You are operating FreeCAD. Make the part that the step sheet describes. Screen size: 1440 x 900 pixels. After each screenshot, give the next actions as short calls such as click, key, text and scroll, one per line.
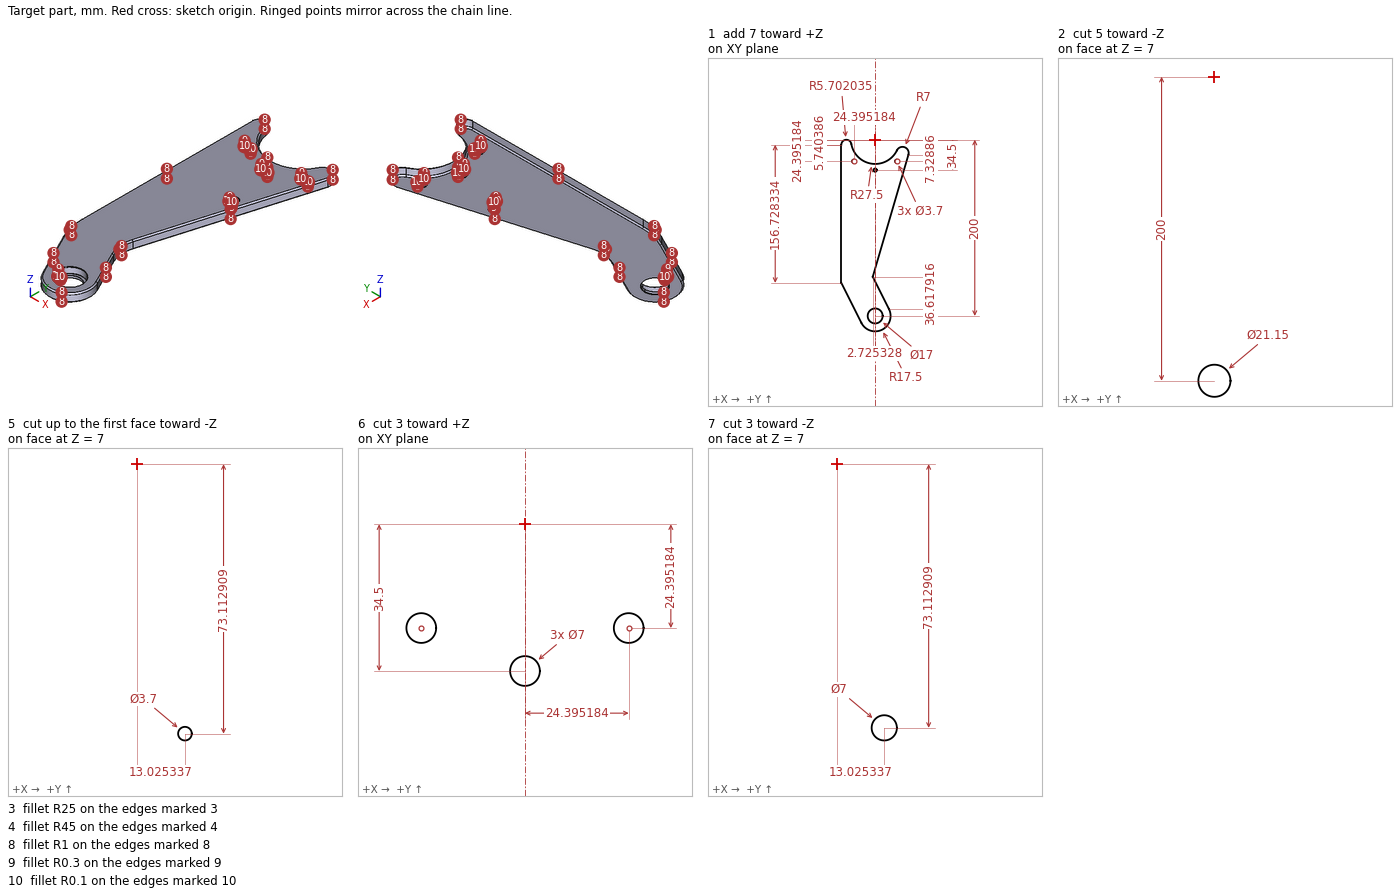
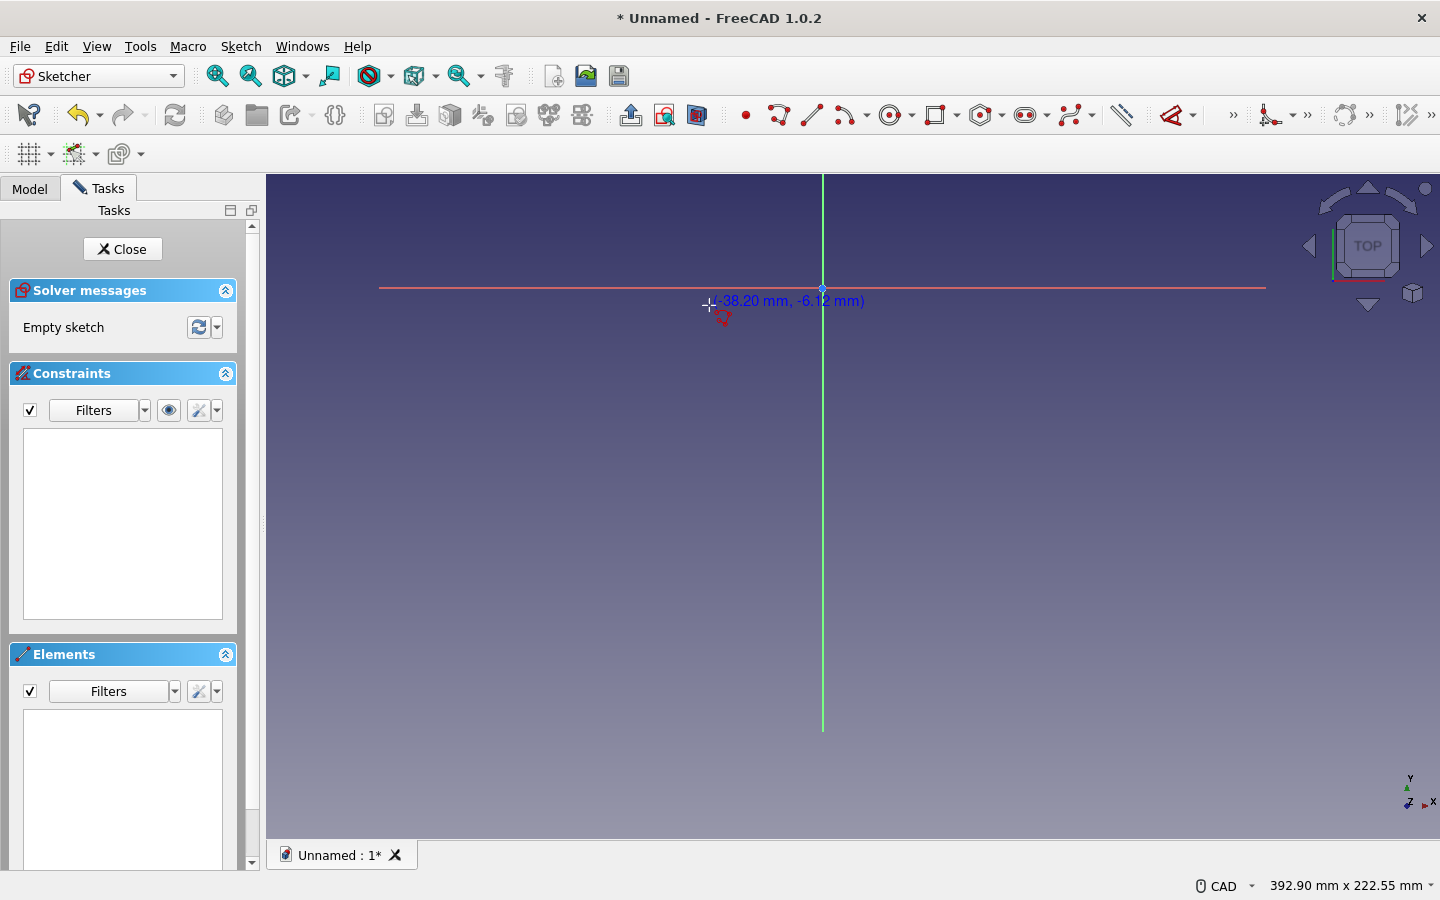
click(708, 305)
click(708, 774)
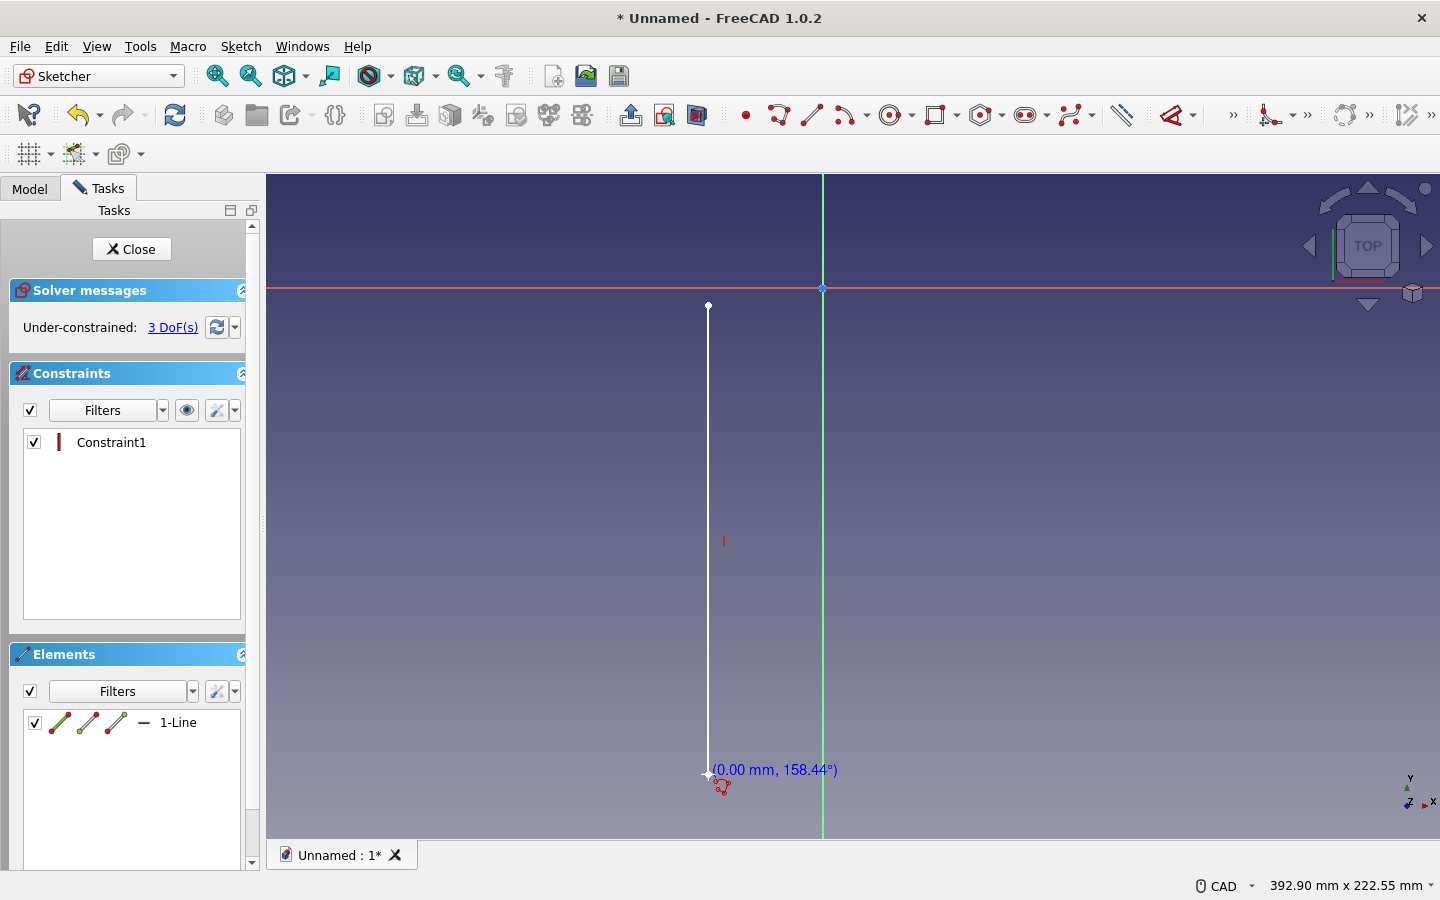
scroll(708, 295, down, 2)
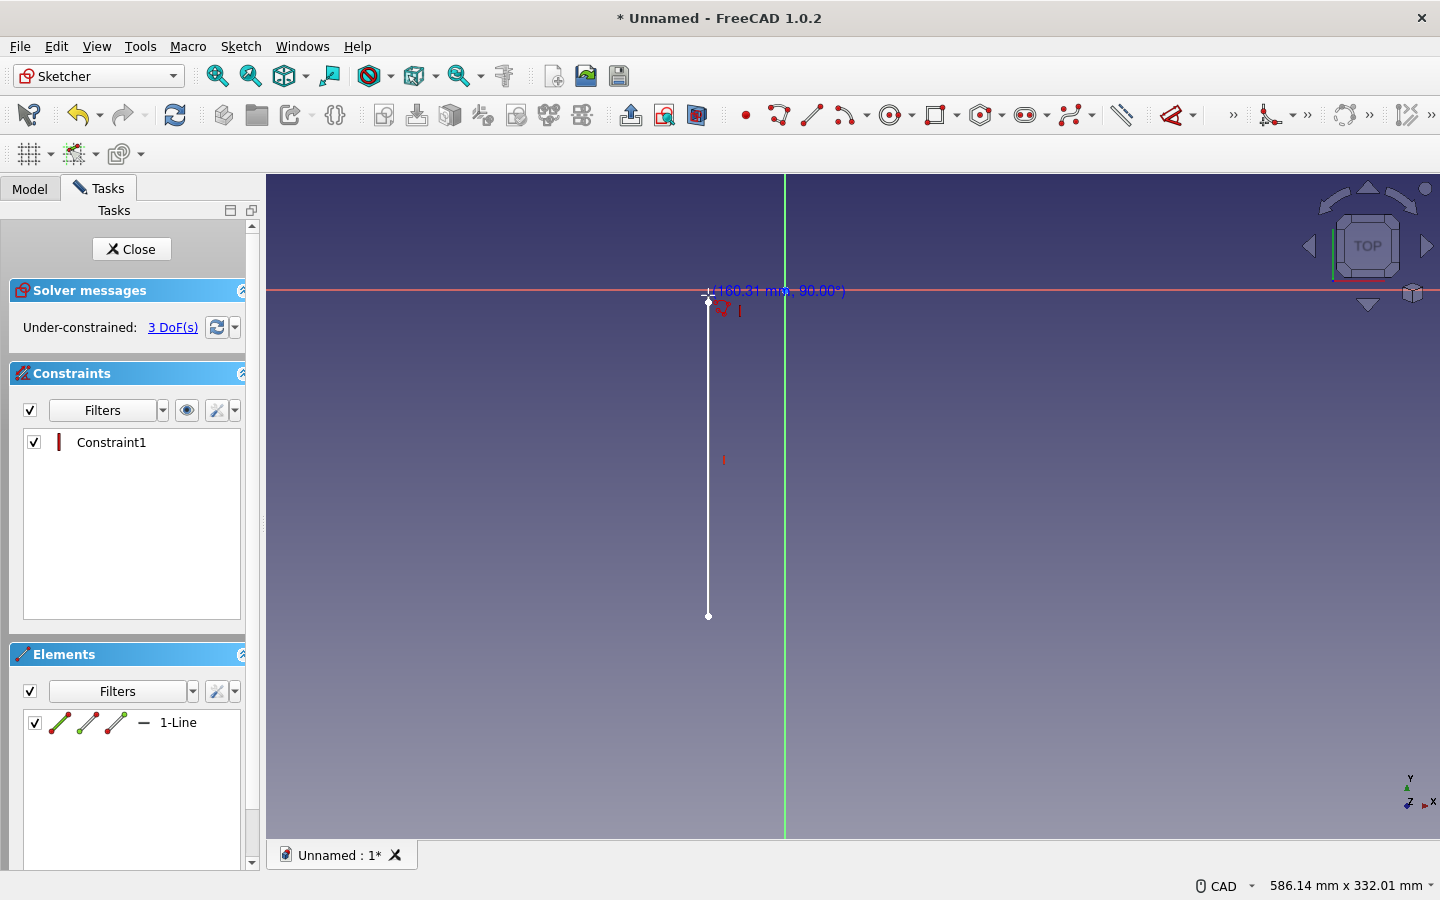
click(754, 707)
right_click(754, 707)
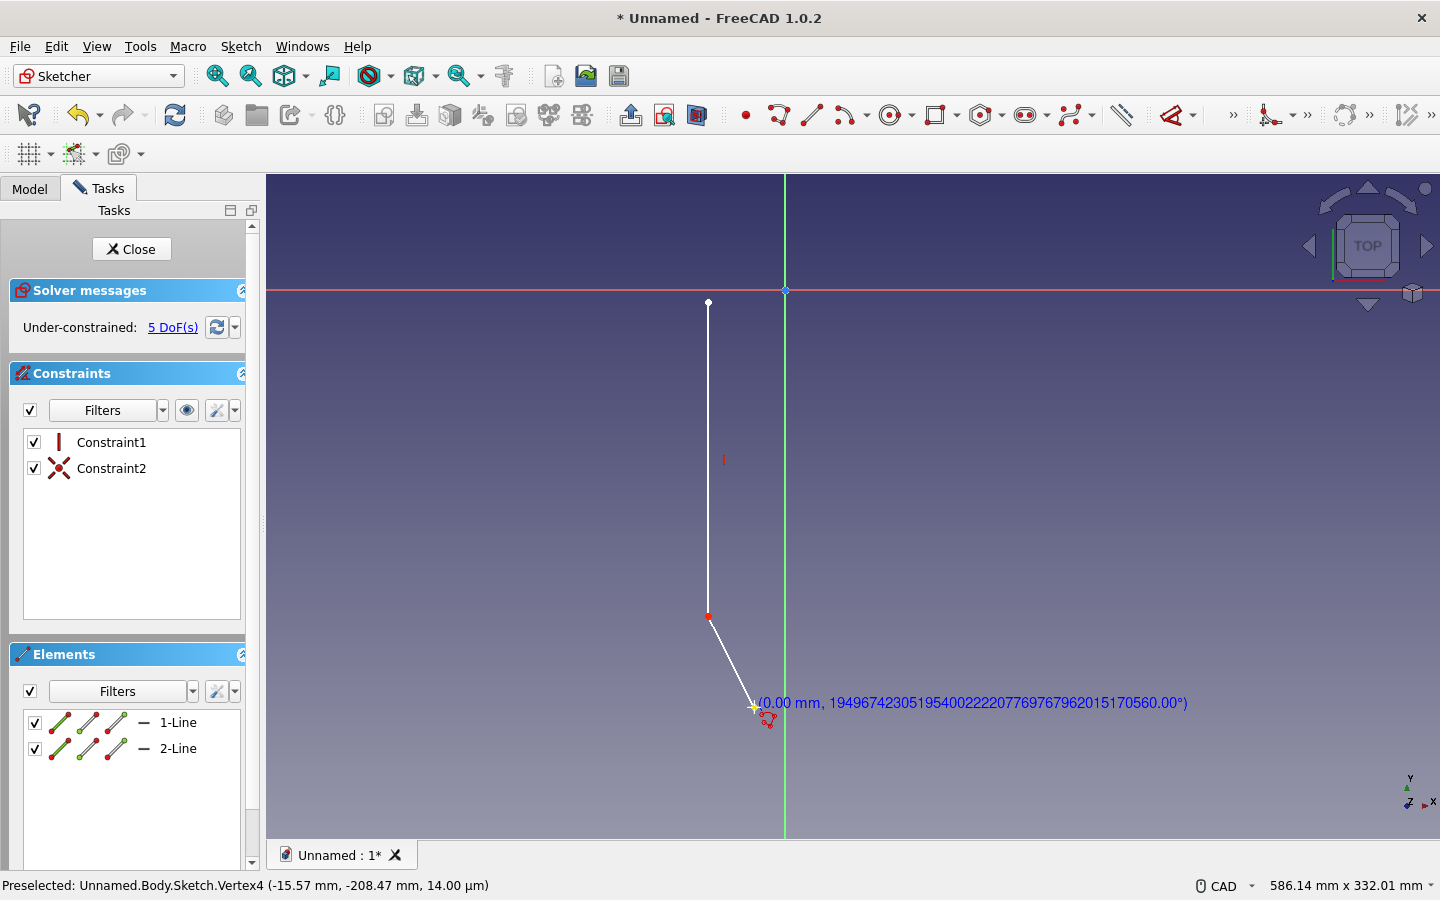
click(817, 675)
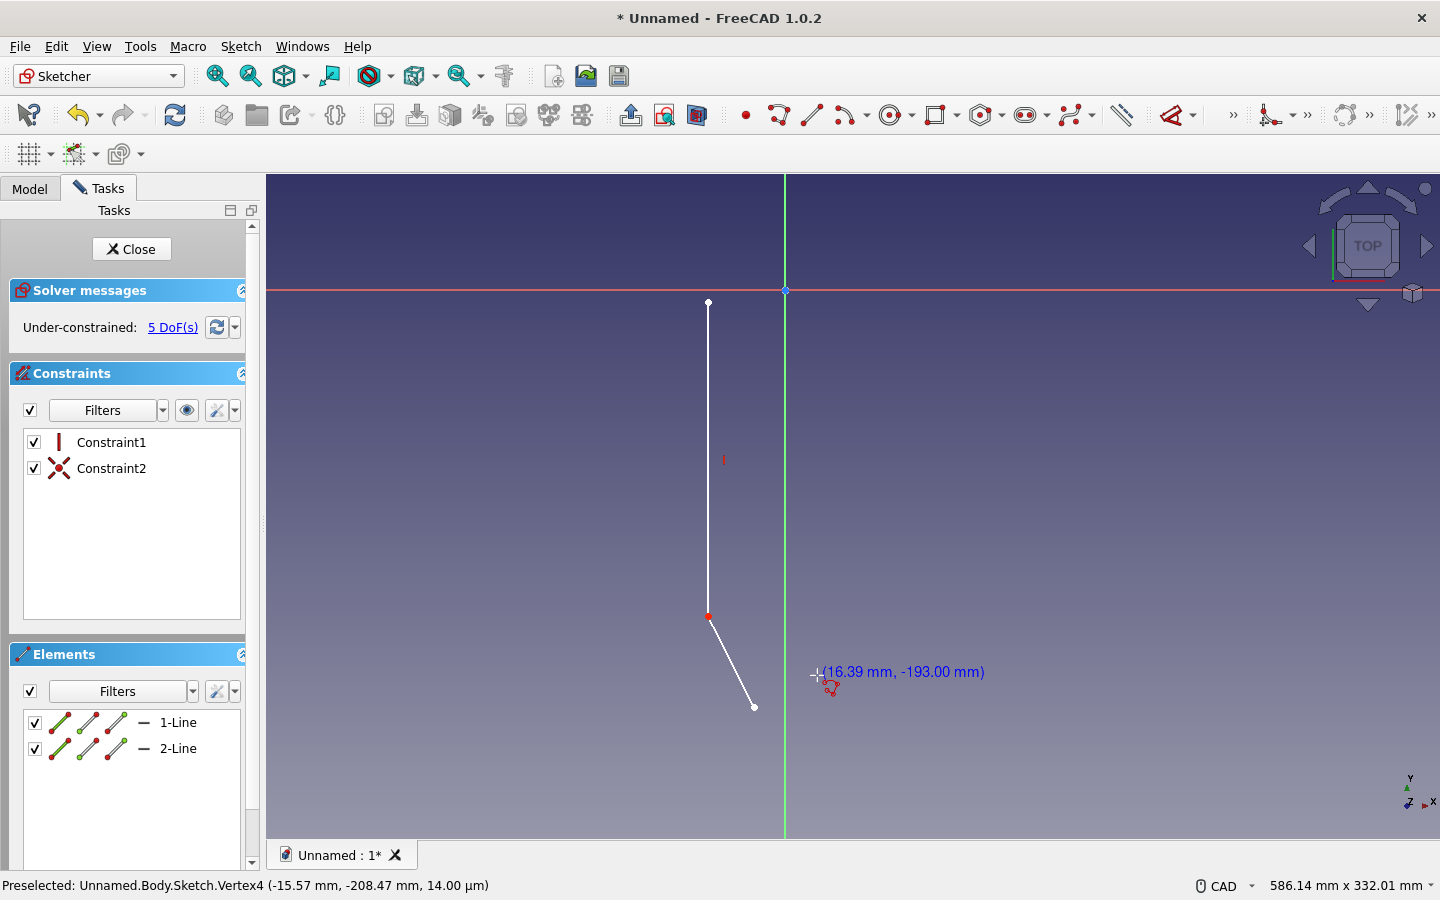
scroll(780, 602, up, 6)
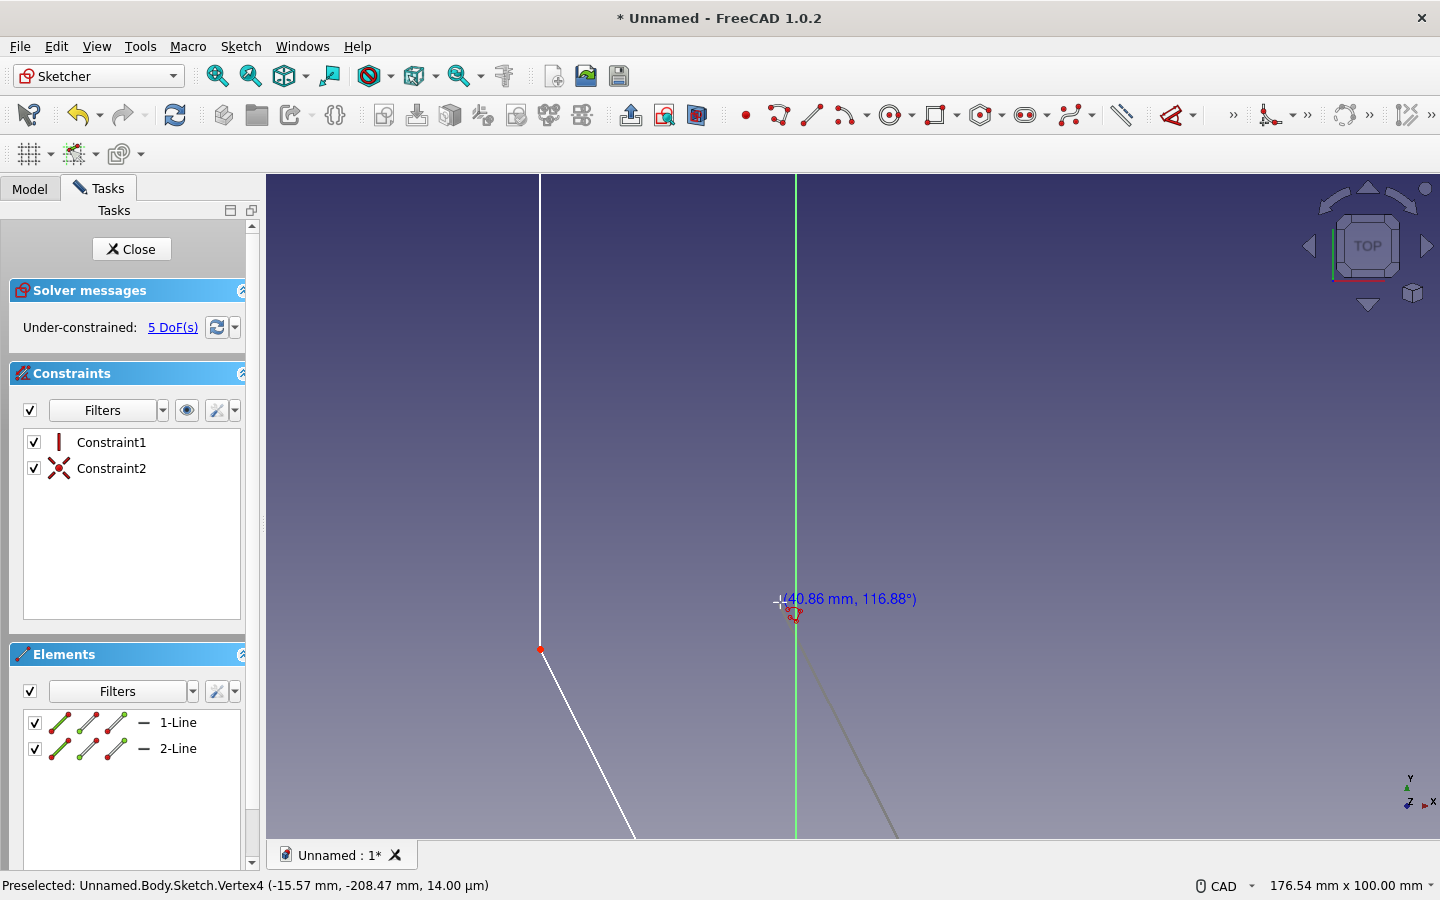
click(778, 600)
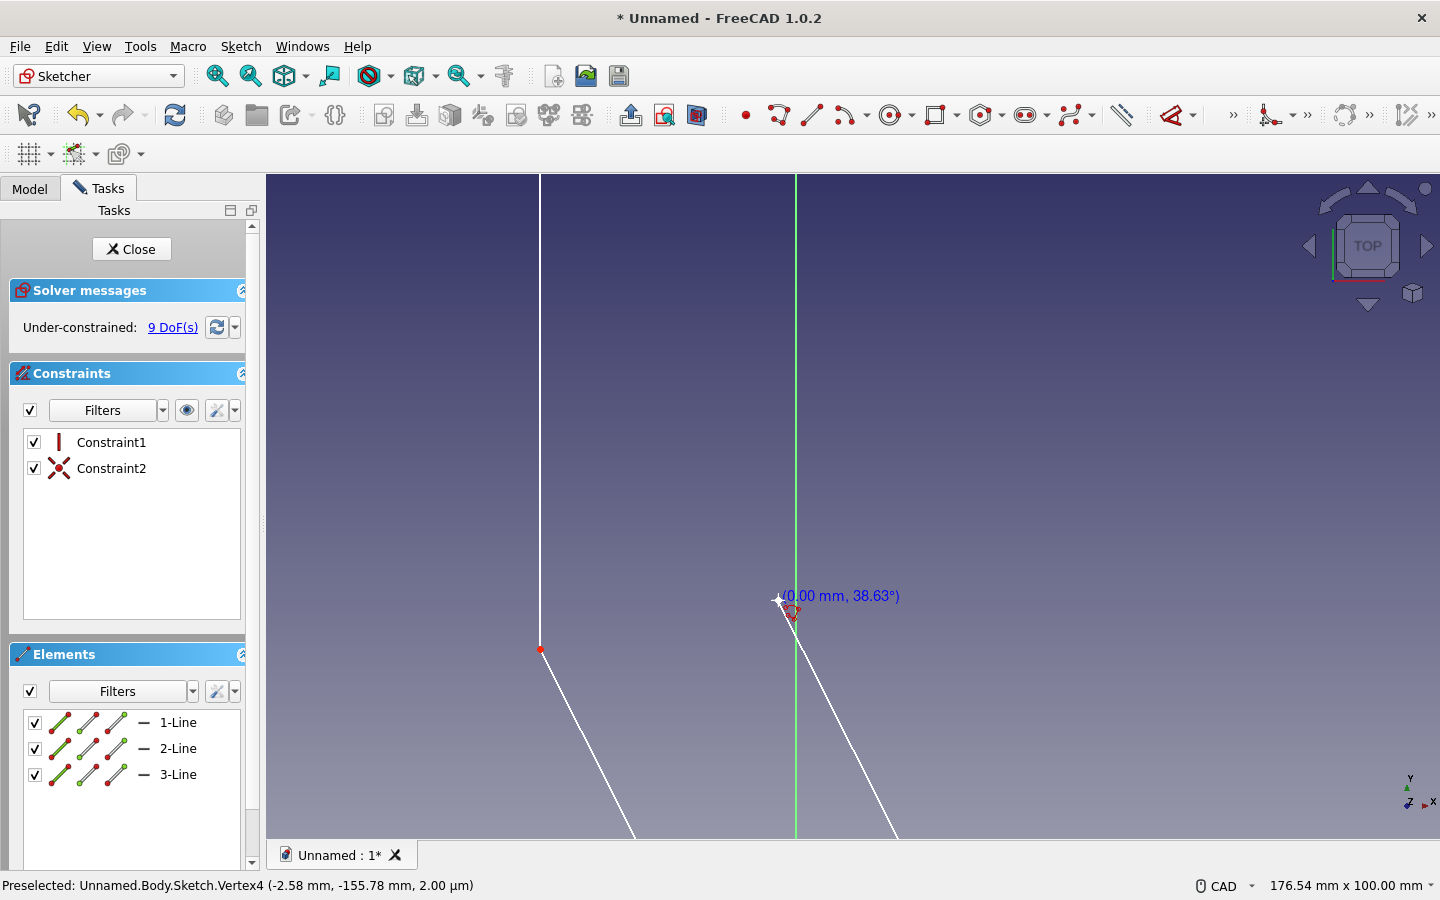
scroll(780, 603, down, 6)